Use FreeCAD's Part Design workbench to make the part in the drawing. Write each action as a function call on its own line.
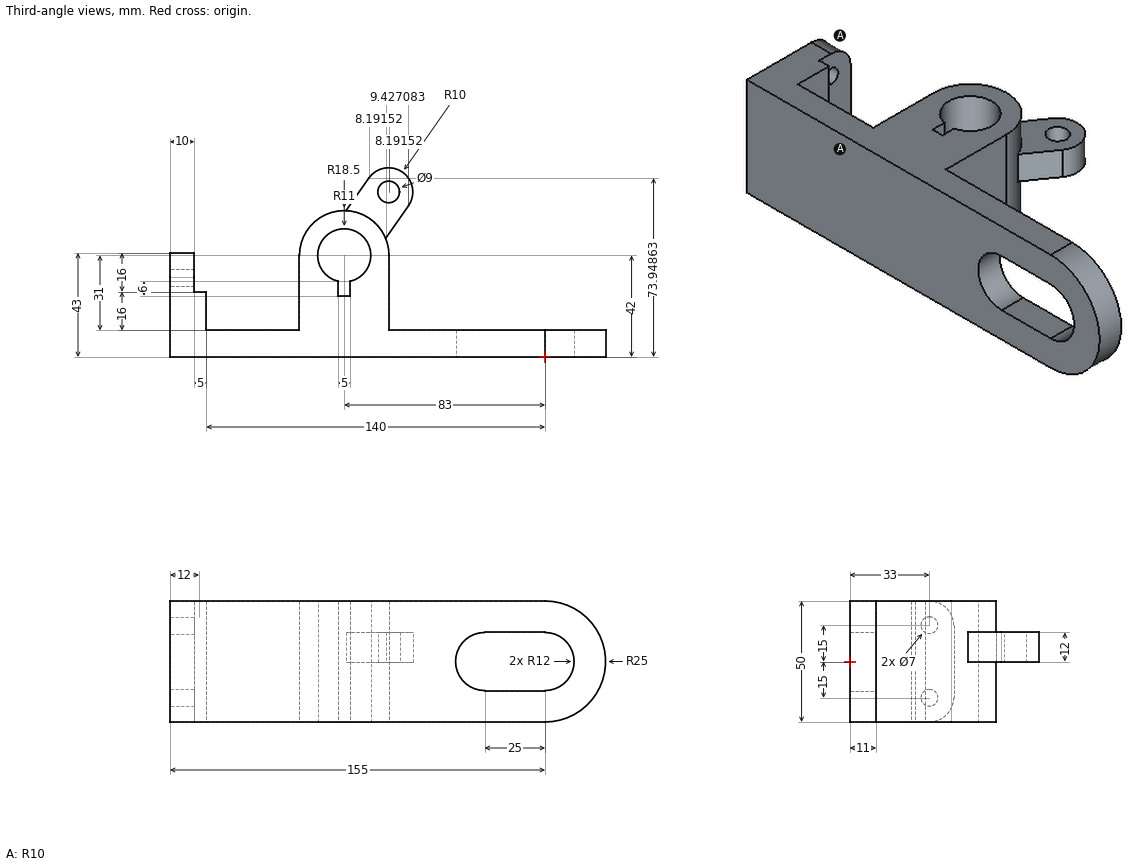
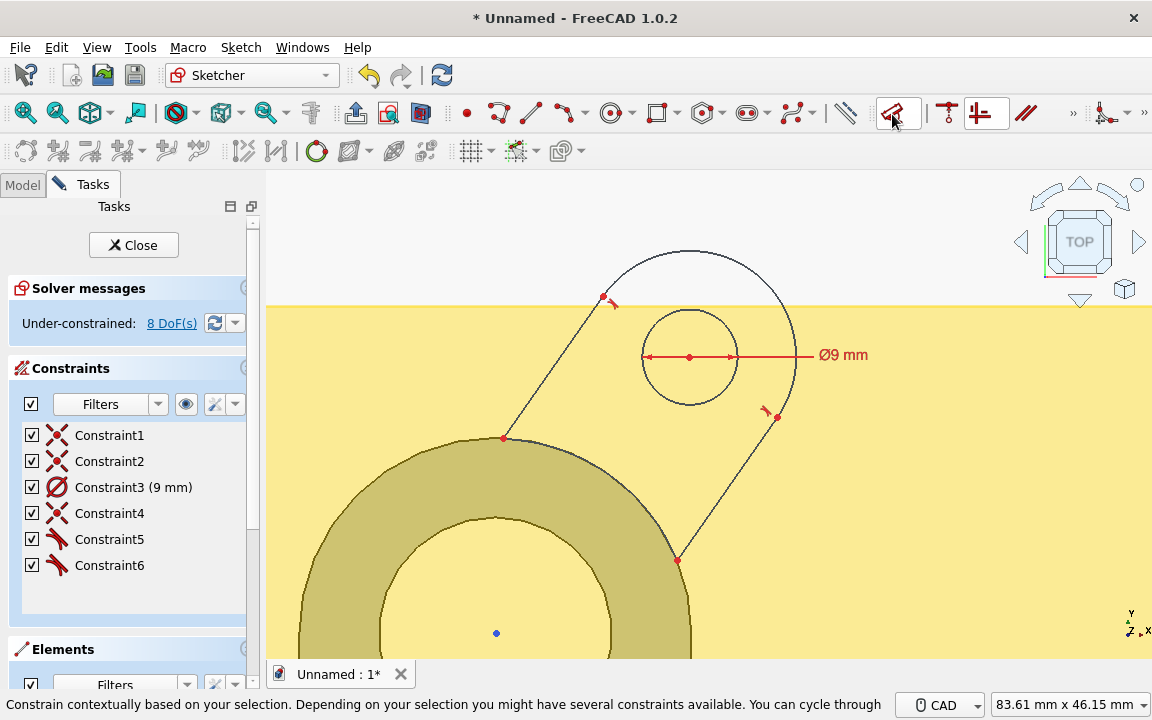
click(790, 323)
click(820, 313)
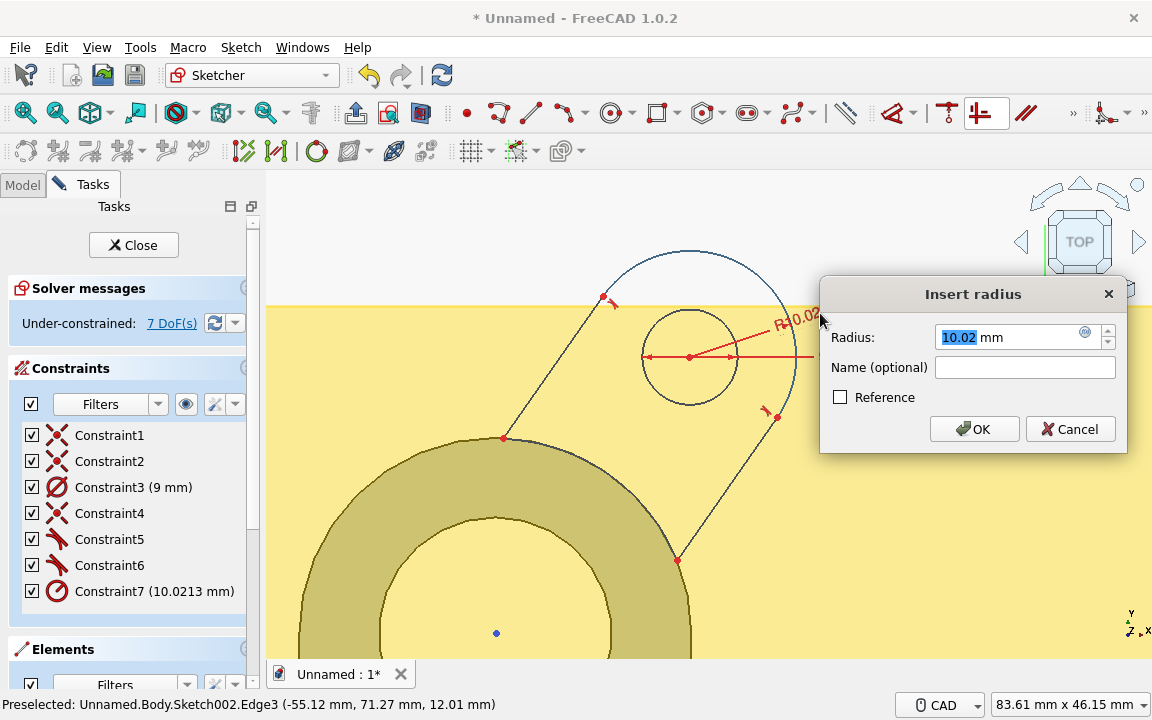
text(10)
key(Return)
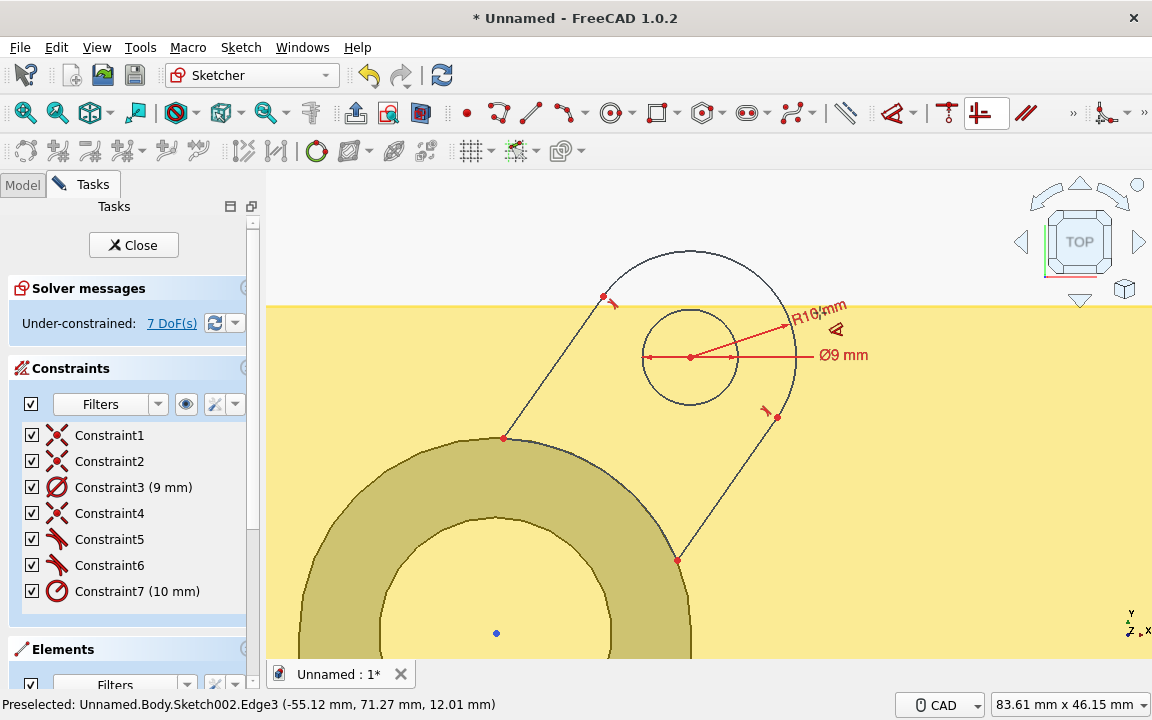
click(642, 504)
click(666, 483)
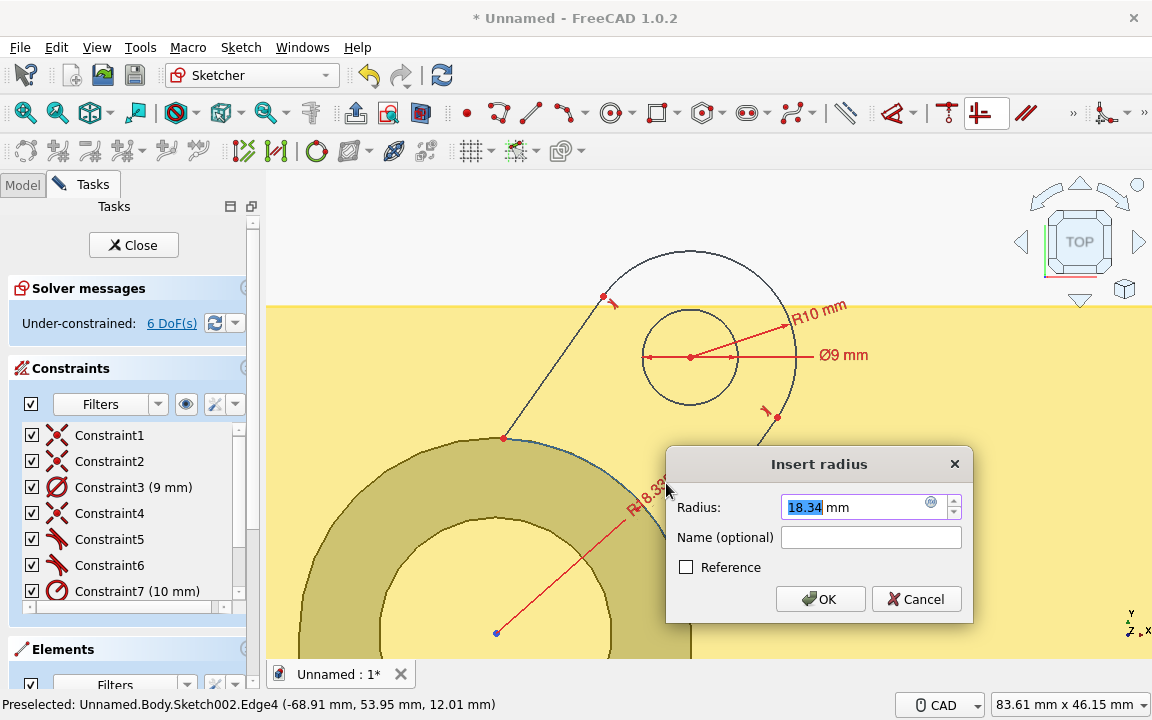
text(18.5)
key(Return)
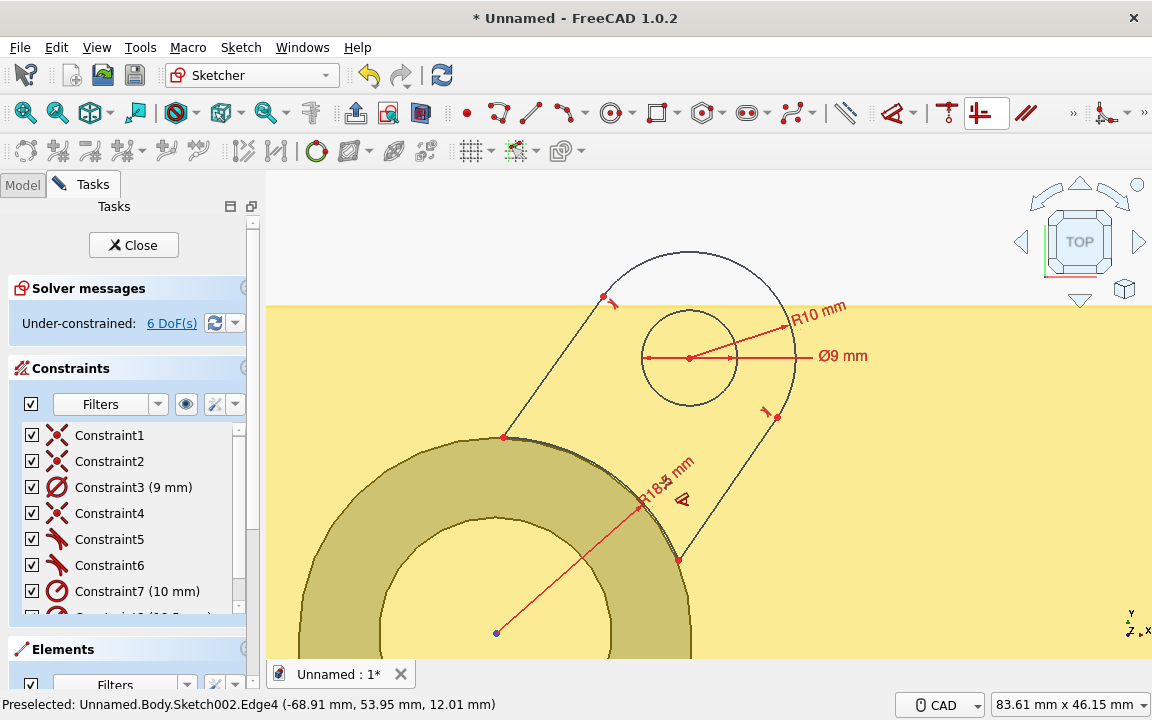
scroll(658, 248, down, 1)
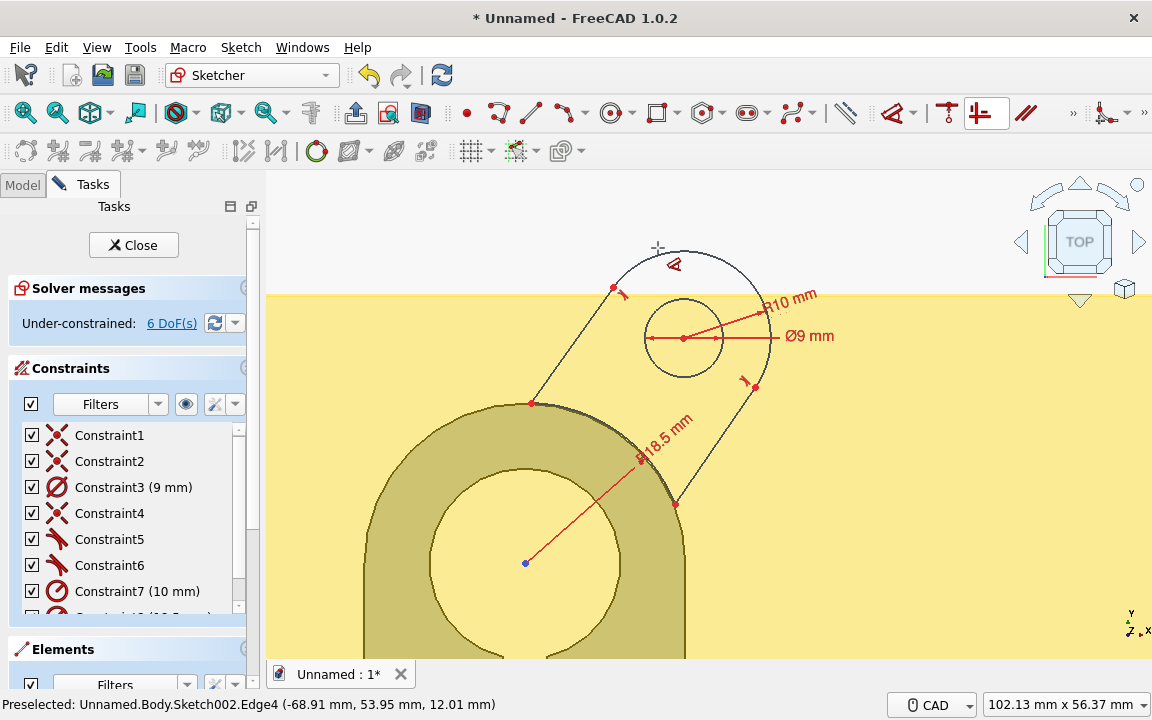
click(526, 563)
click(756, 529)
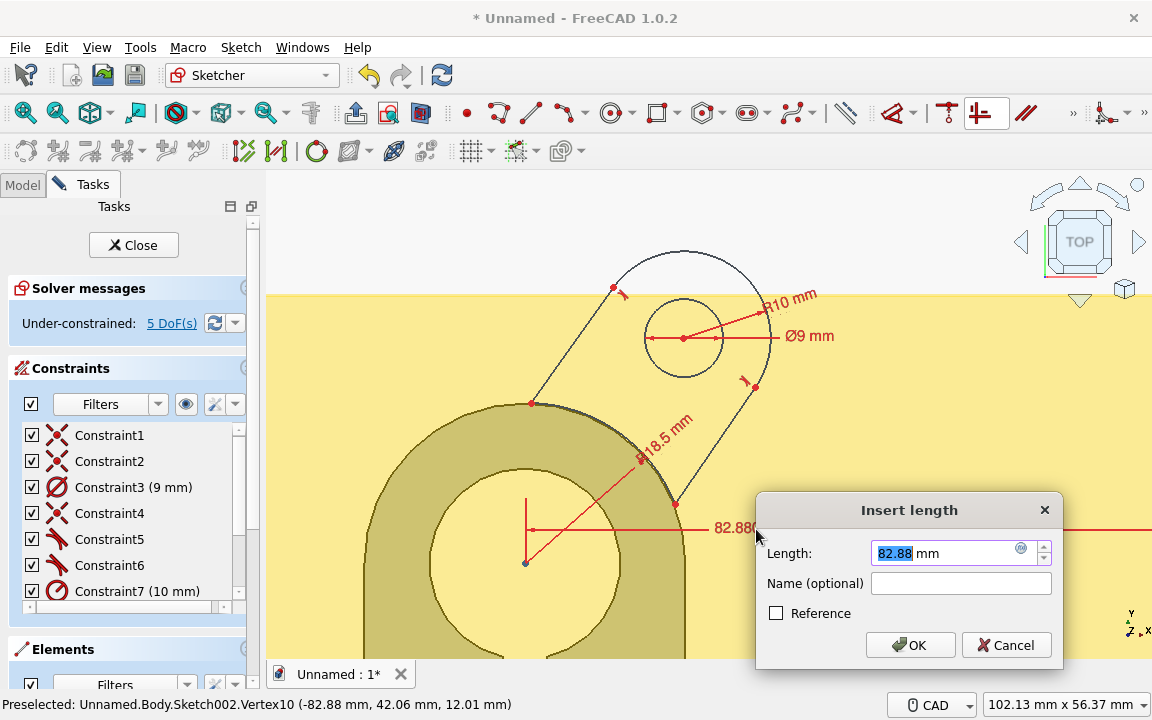
text(83)
key(Return)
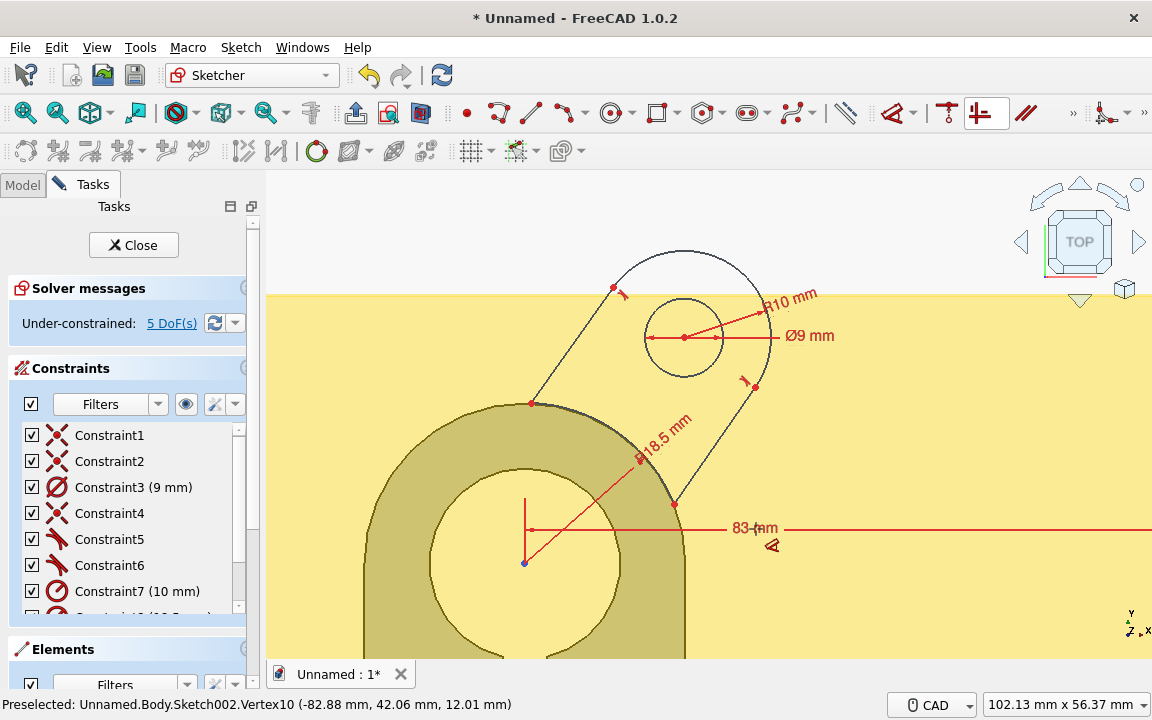
click(525, 563)
click(491, 597)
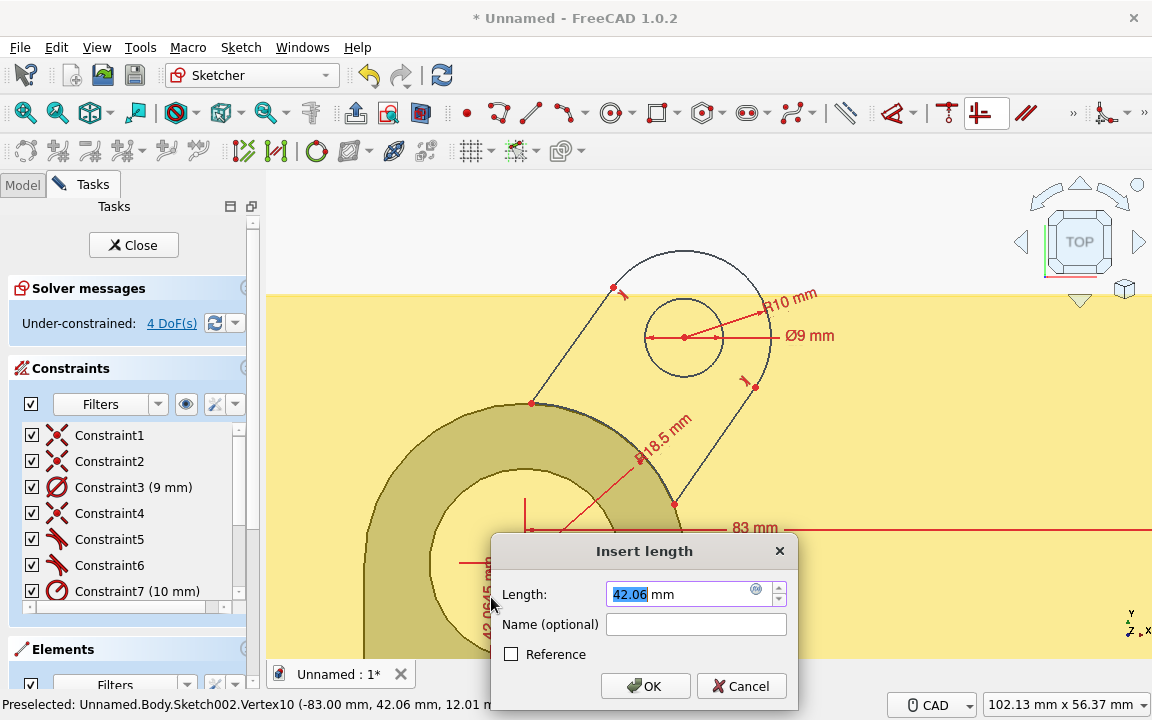
text(42)
key(Return)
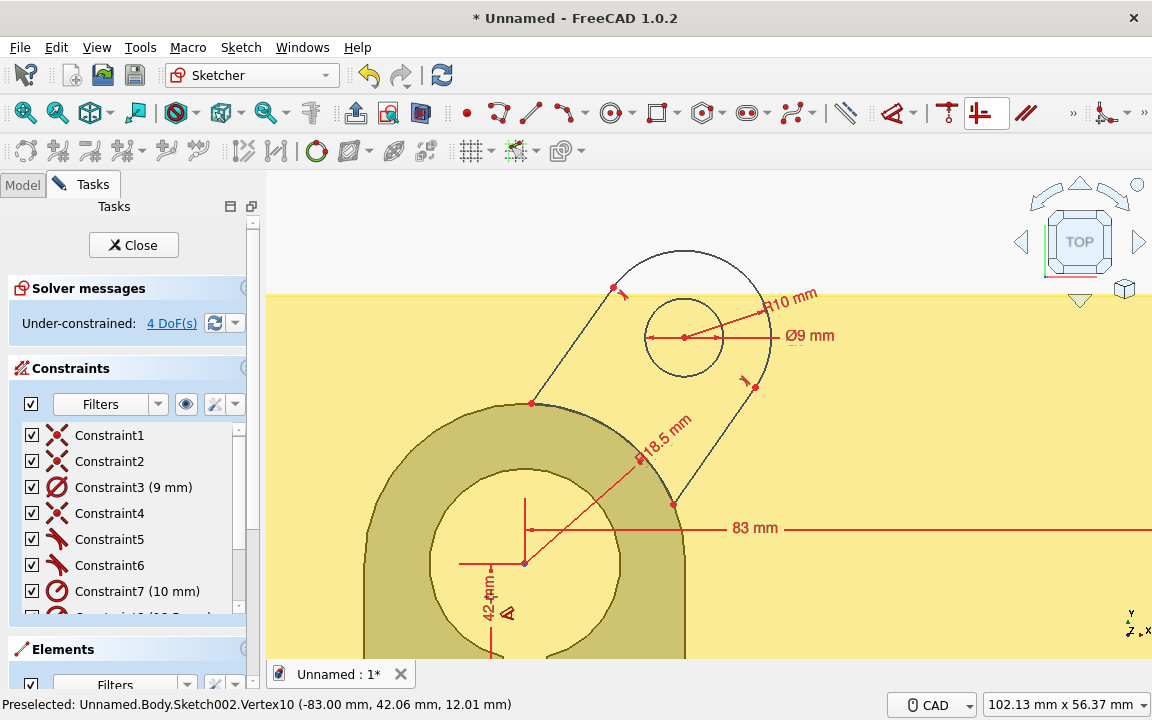
click(755, 387)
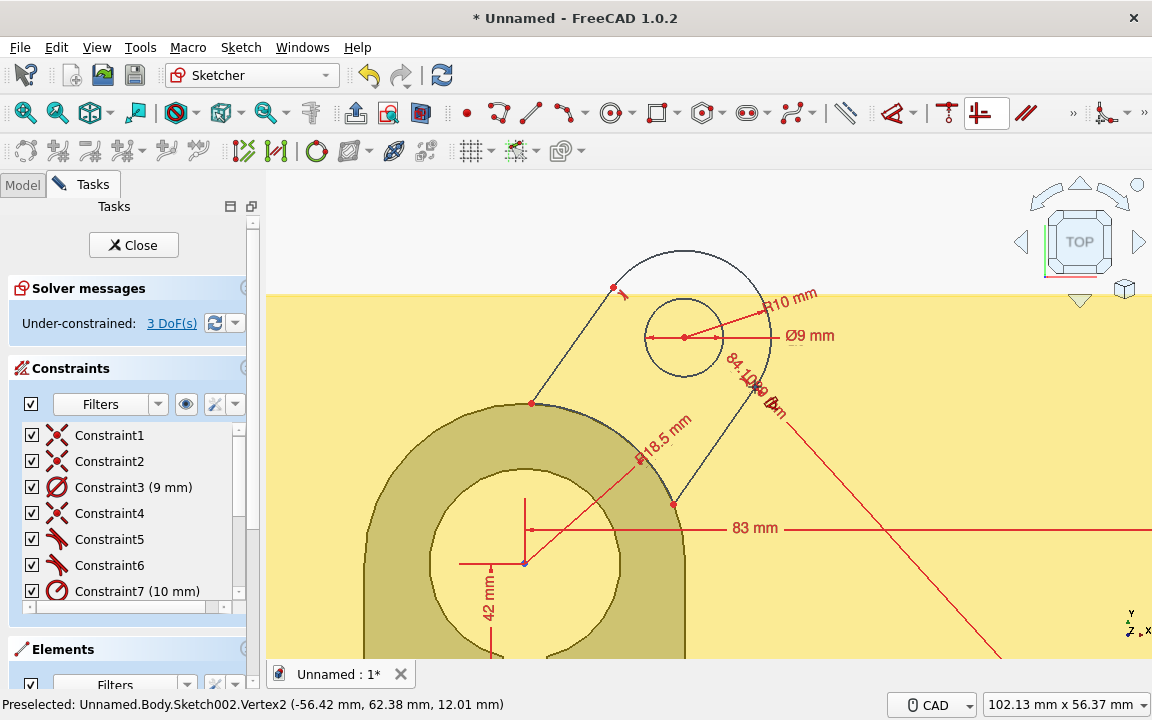
click(684, 338)
click(720, 280)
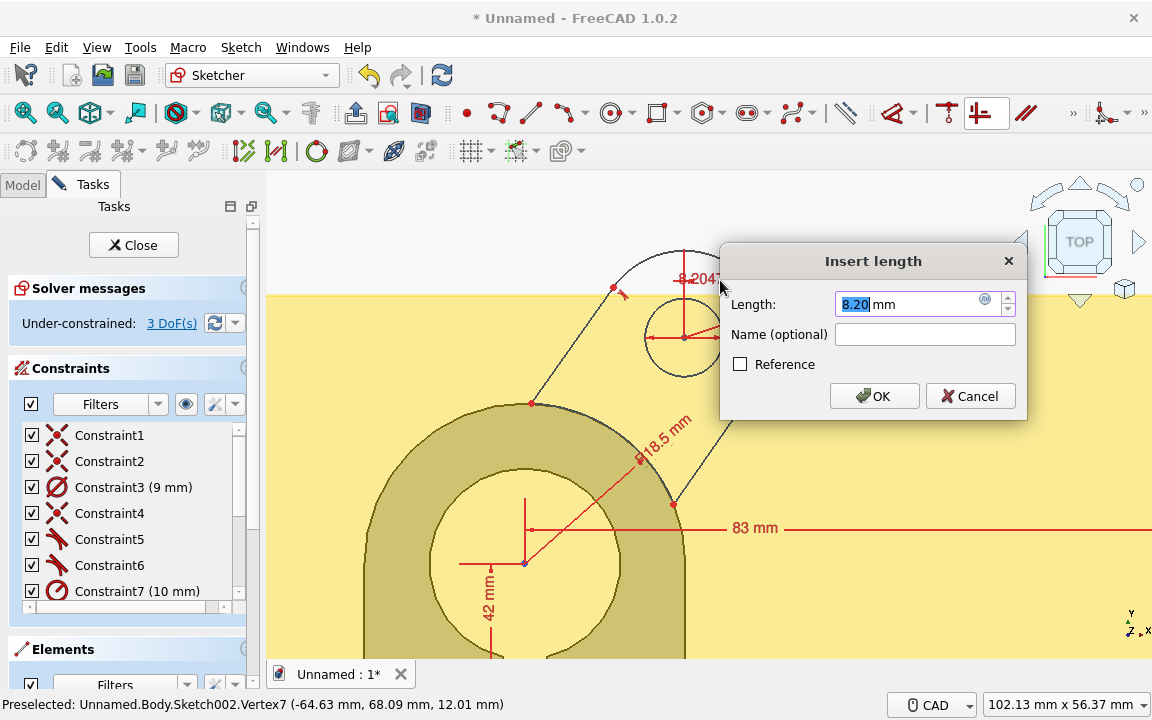
text(8.19152)
key(Return)